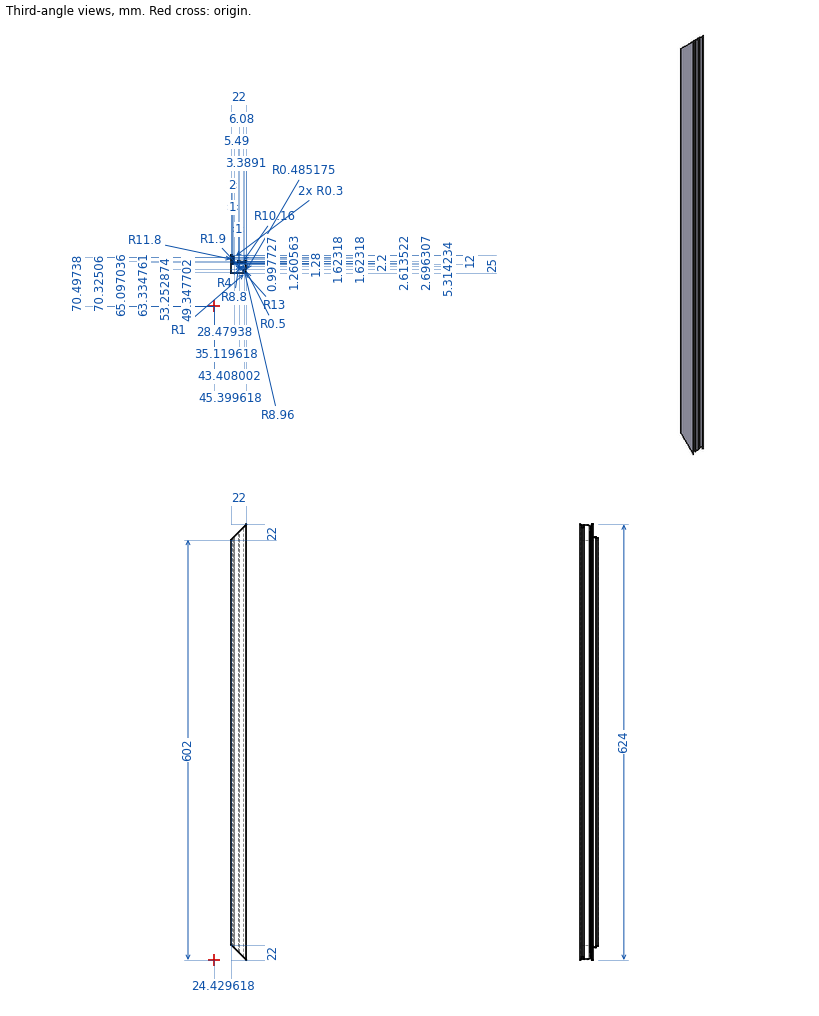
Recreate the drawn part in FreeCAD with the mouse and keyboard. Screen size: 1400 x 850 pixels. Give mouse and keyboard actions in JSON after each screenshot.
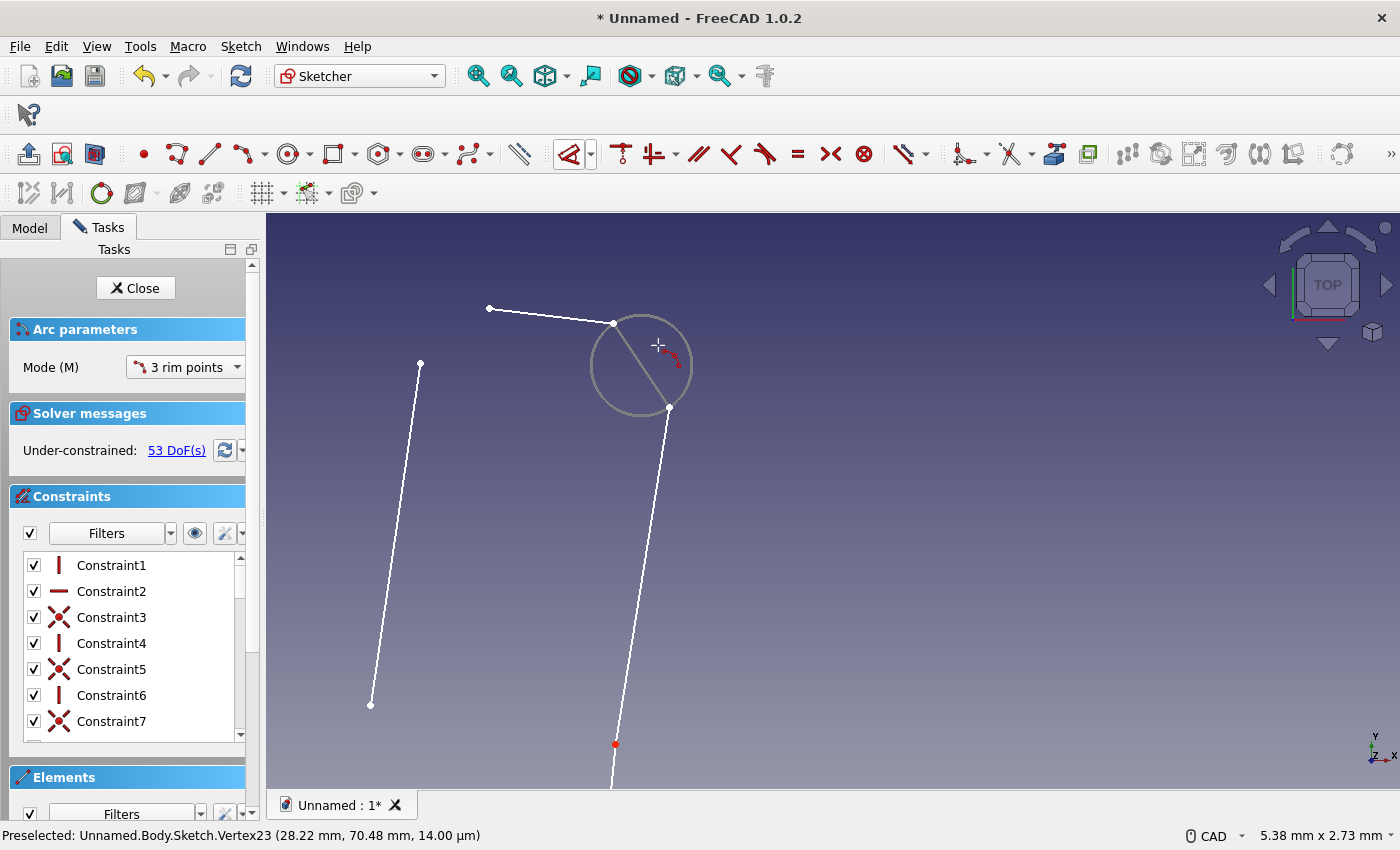
{"action": "left_click", "coordinate": [656, 345]}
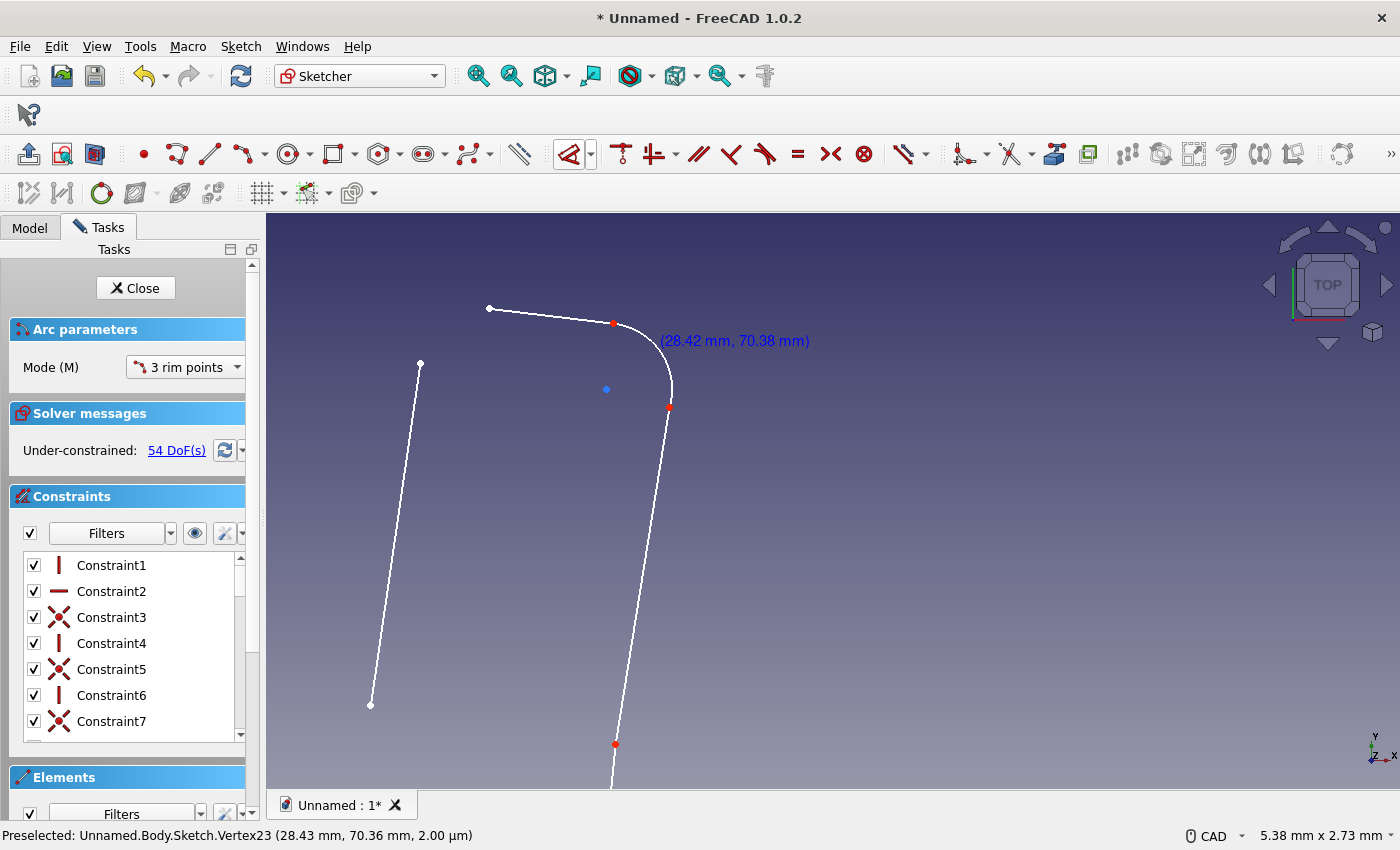
{"action": "scroll", "coordinate": [655, 350], "scroll_direction": "down", "scroll_amount": 13}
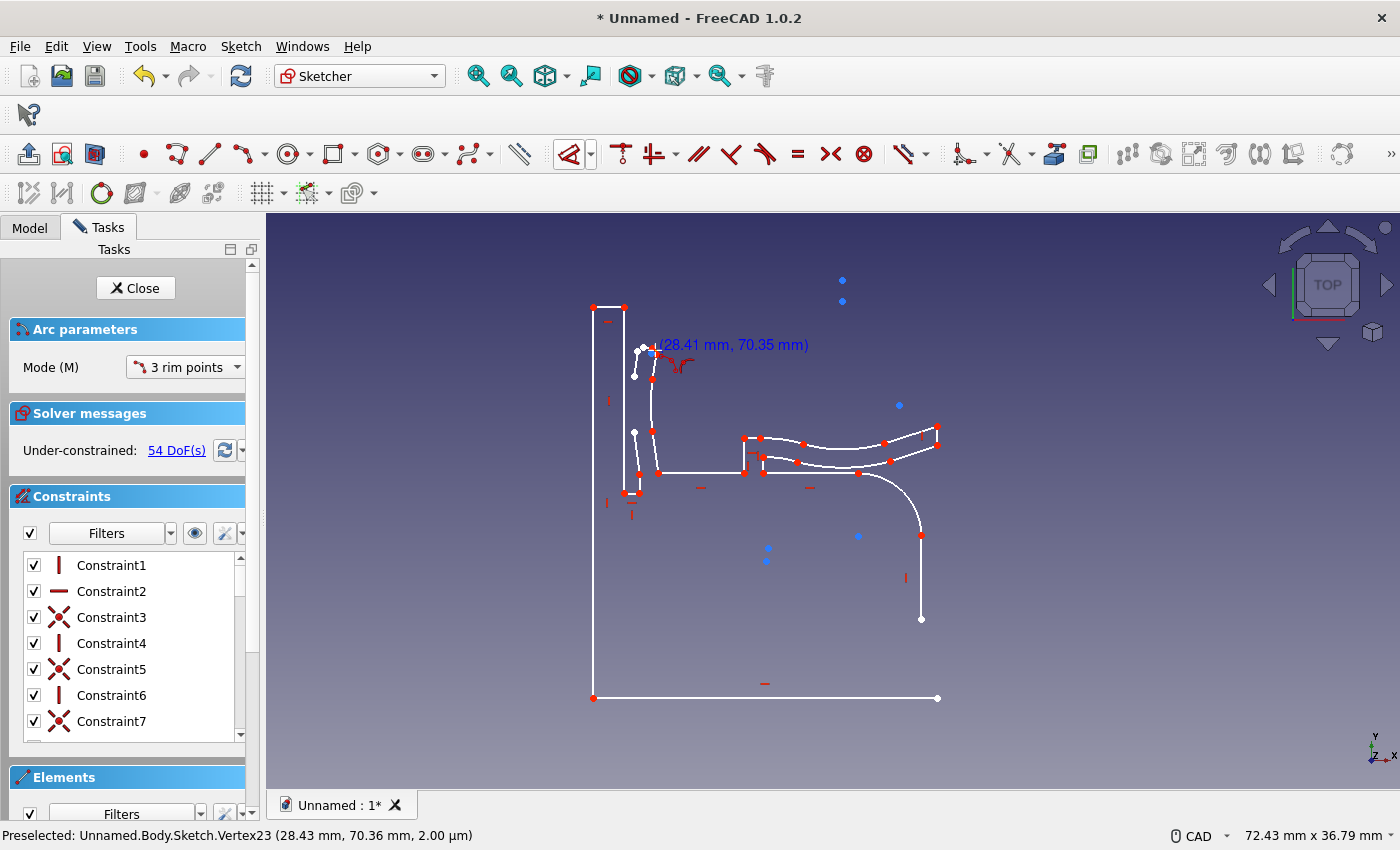
{"action": "scroll", "coordinate": [643, 347], "scroll_direction": "up", "scroll_amount": 7}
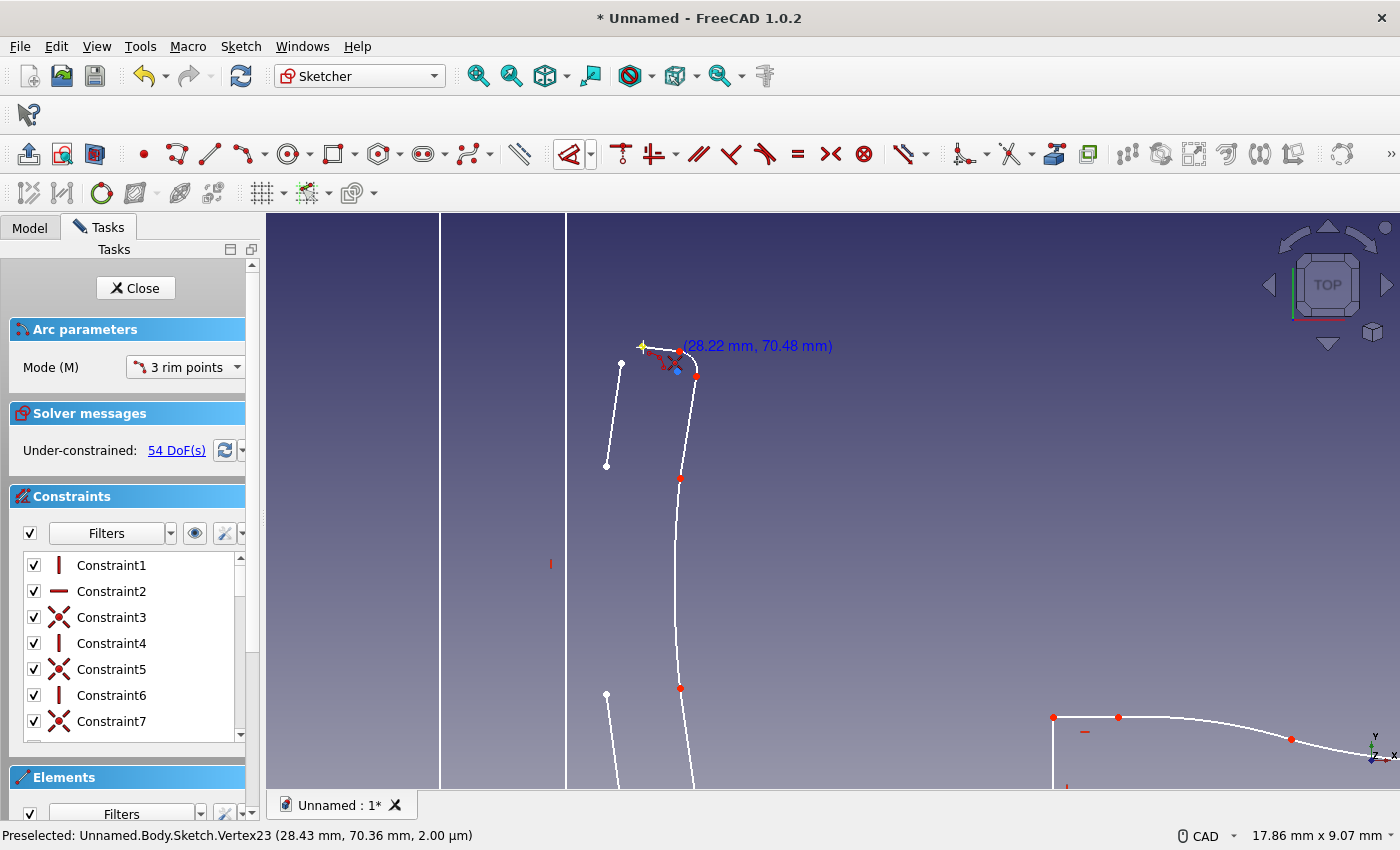
{"action": "left_click", "coordinate": [642, 347]}
{"action": "left_click", "coordinate": [621, 363]}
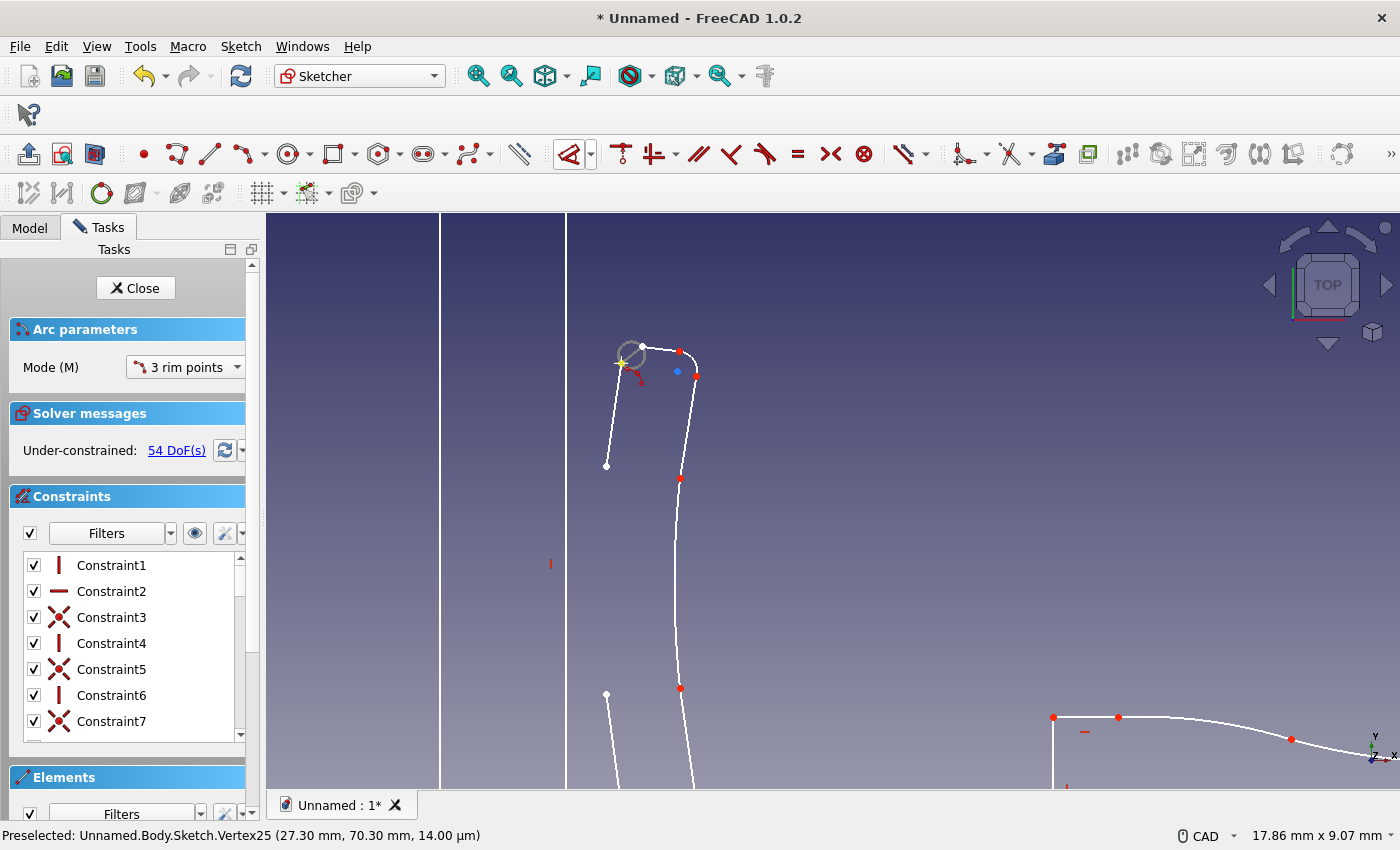
{"action": "scroll", "coordinate": [628, 349], "scroll_direction": "up", "scroll_amount": 6}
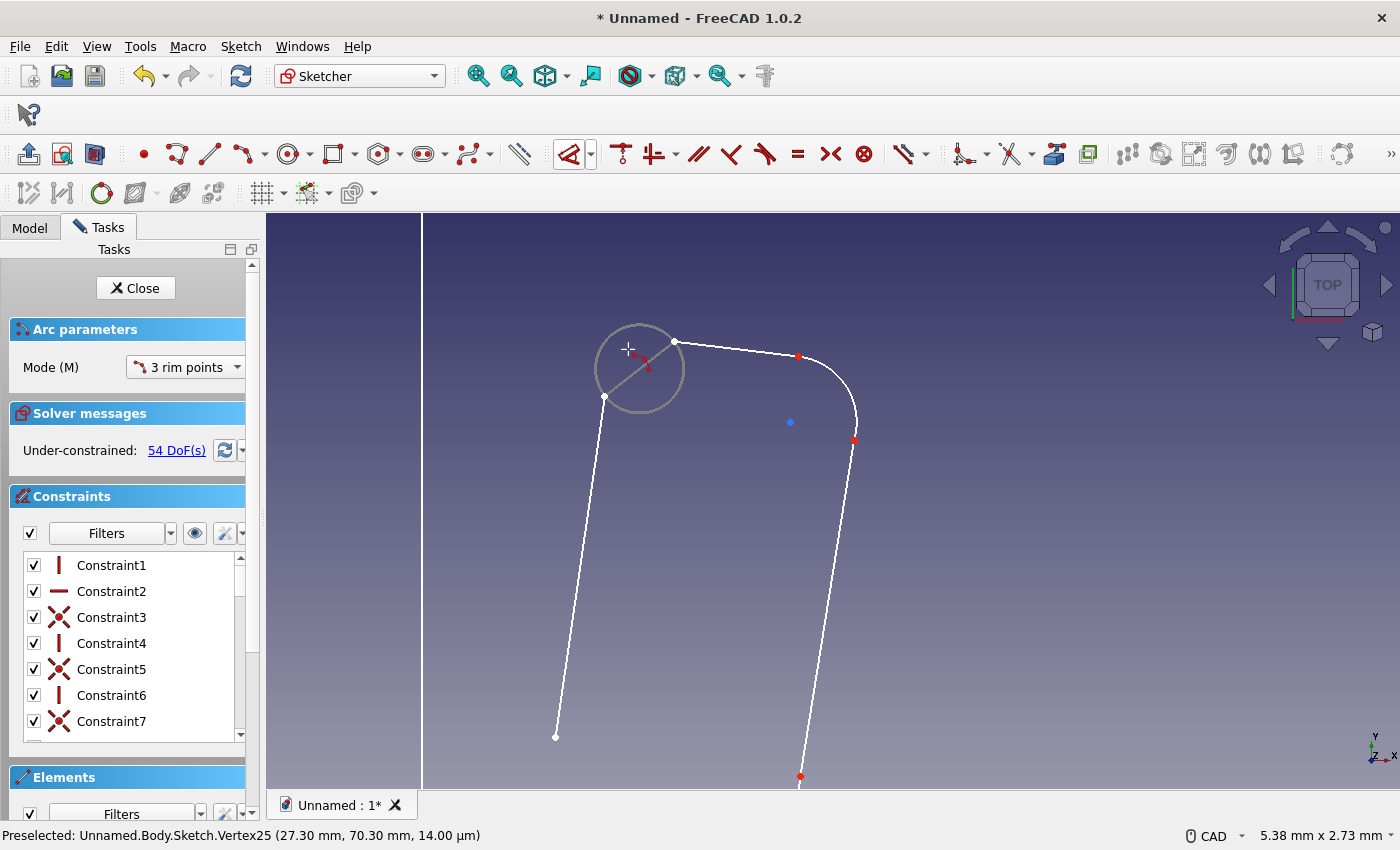
{"action": "left_click", "coordinate": [627, 348]}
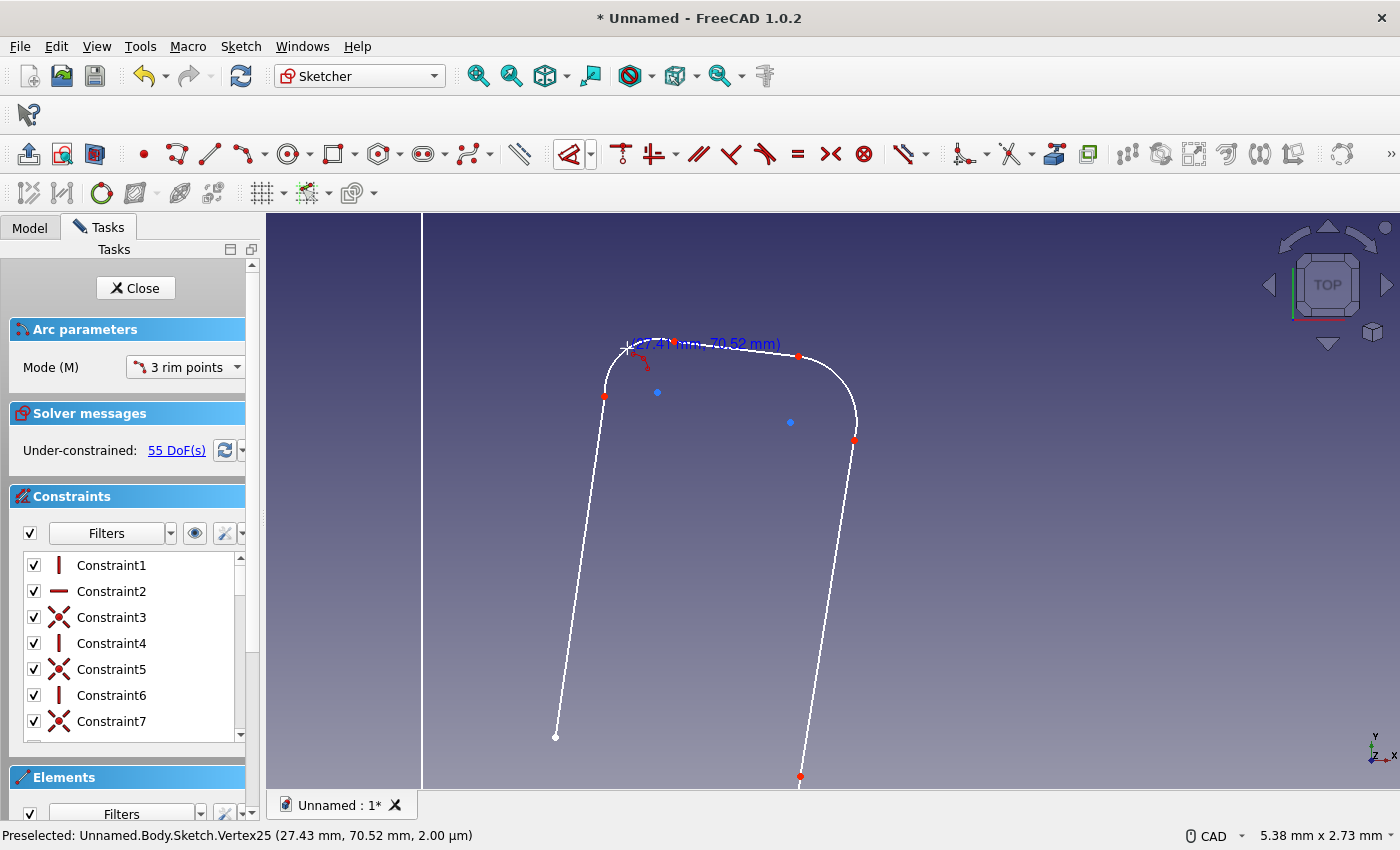
{"action": "scroll", "coordinate": [640, 347], "scroll_direction": "down", "scroll_amount": 13}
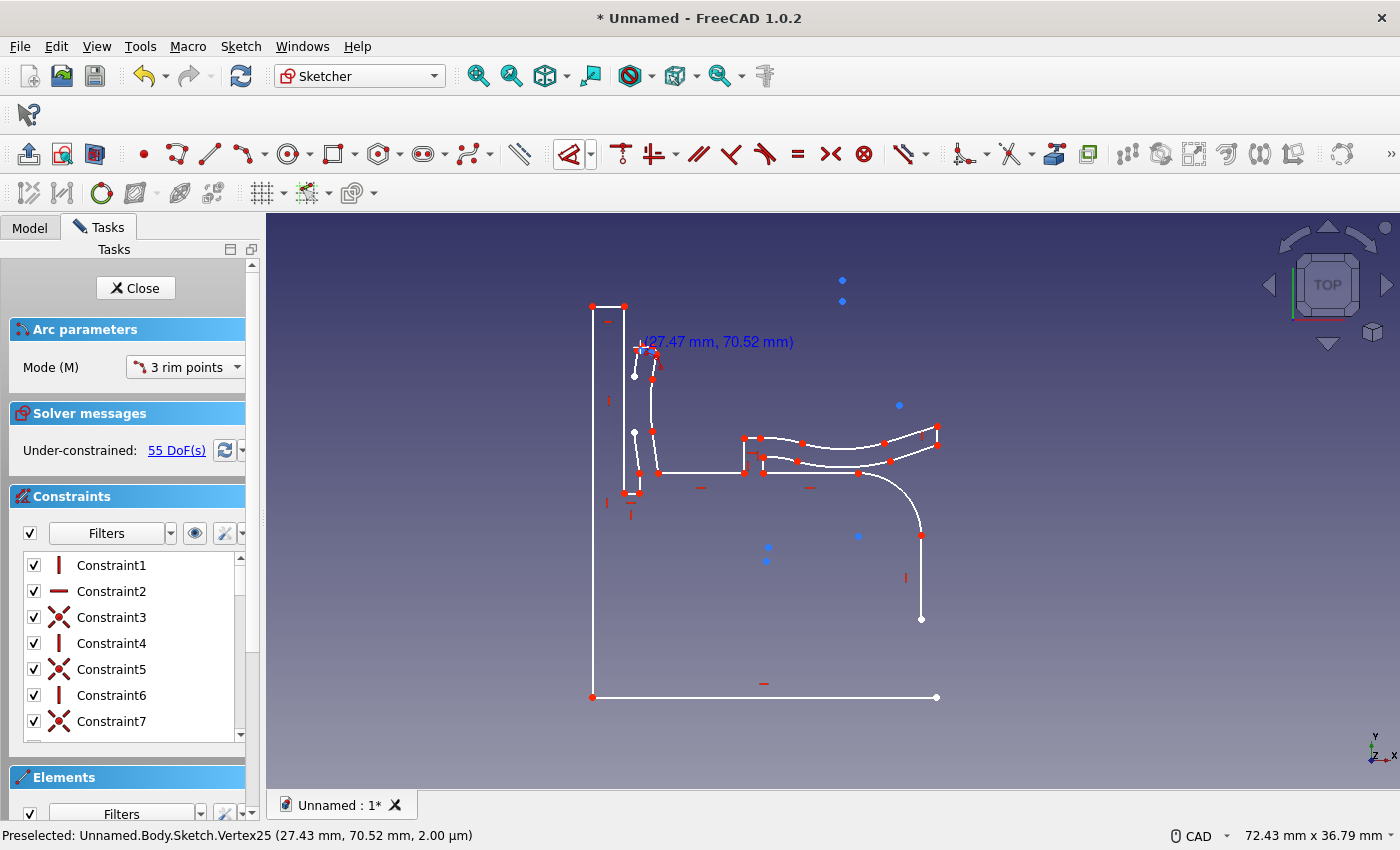
{"action": "scroll", "coordinate": [634, 376], "scroll_direction": "up", "scroll_amount": 3}